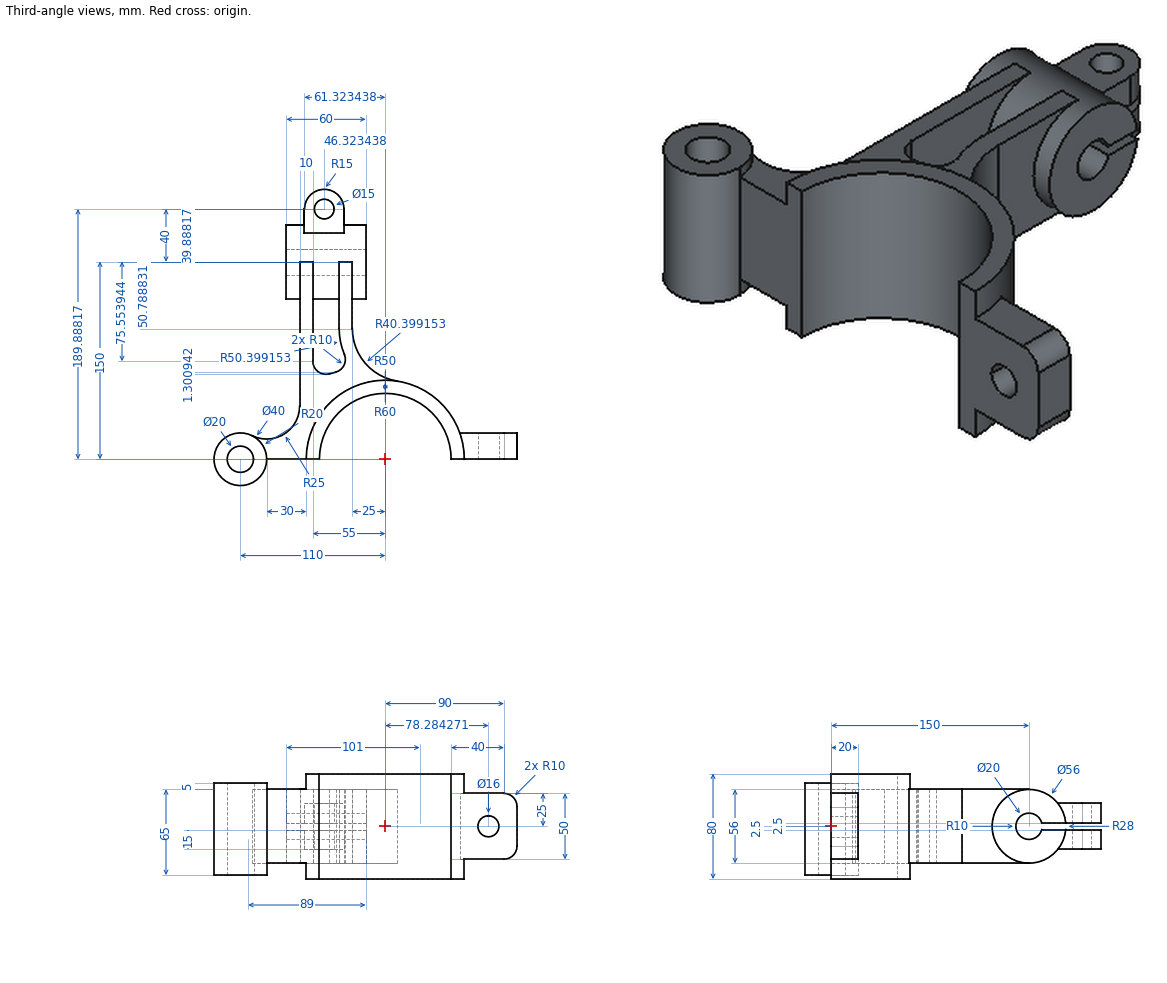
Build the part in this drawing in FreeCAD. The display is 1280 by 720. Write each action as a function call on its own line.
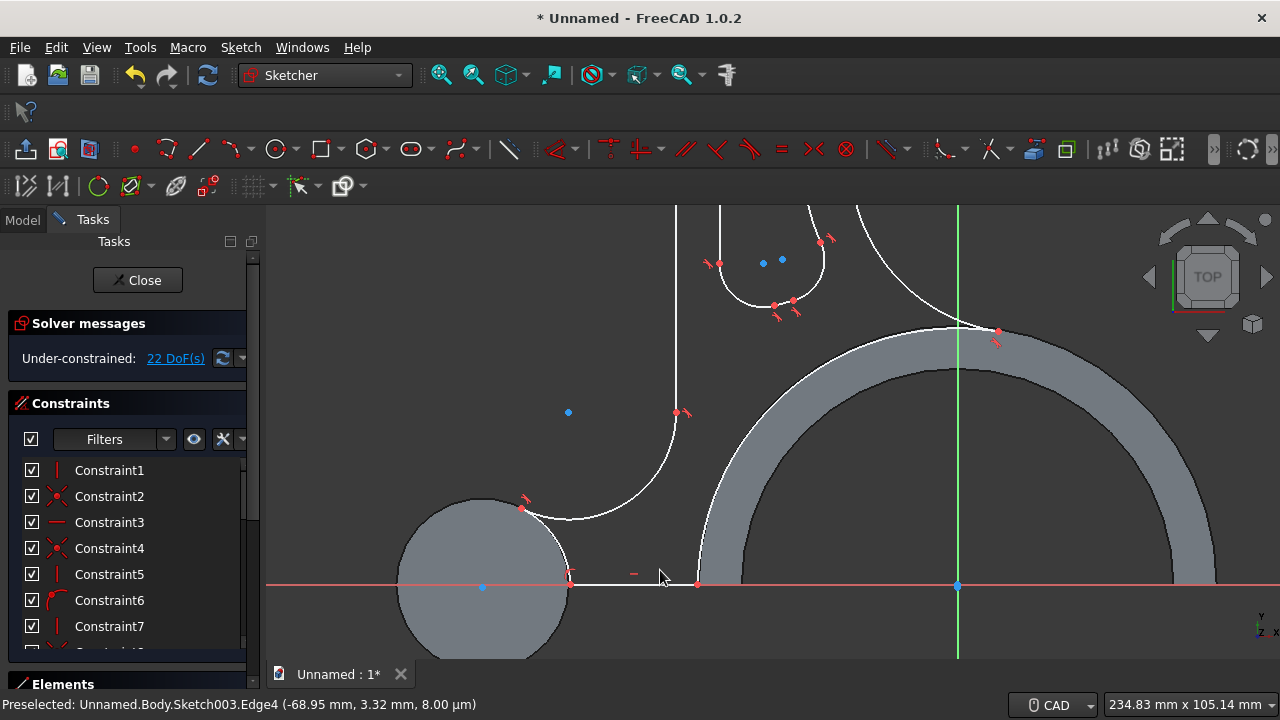
click(929, 305)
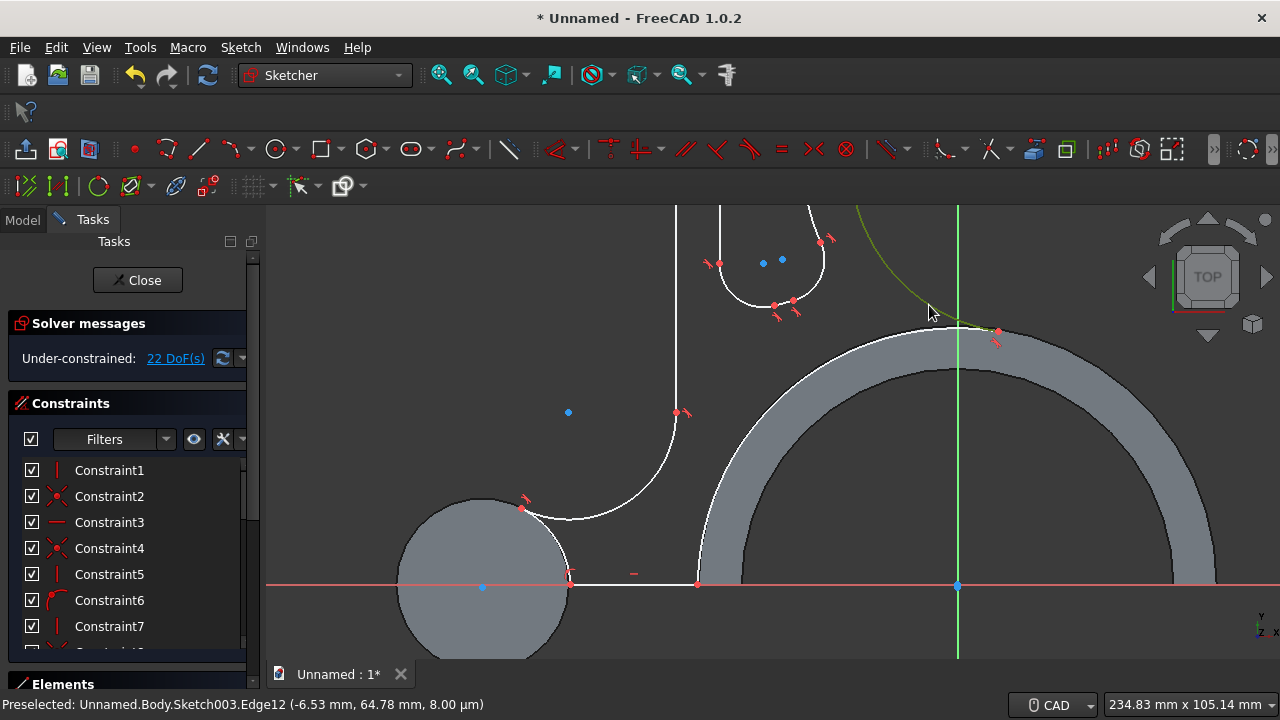
scroll(660, 572, down, 4)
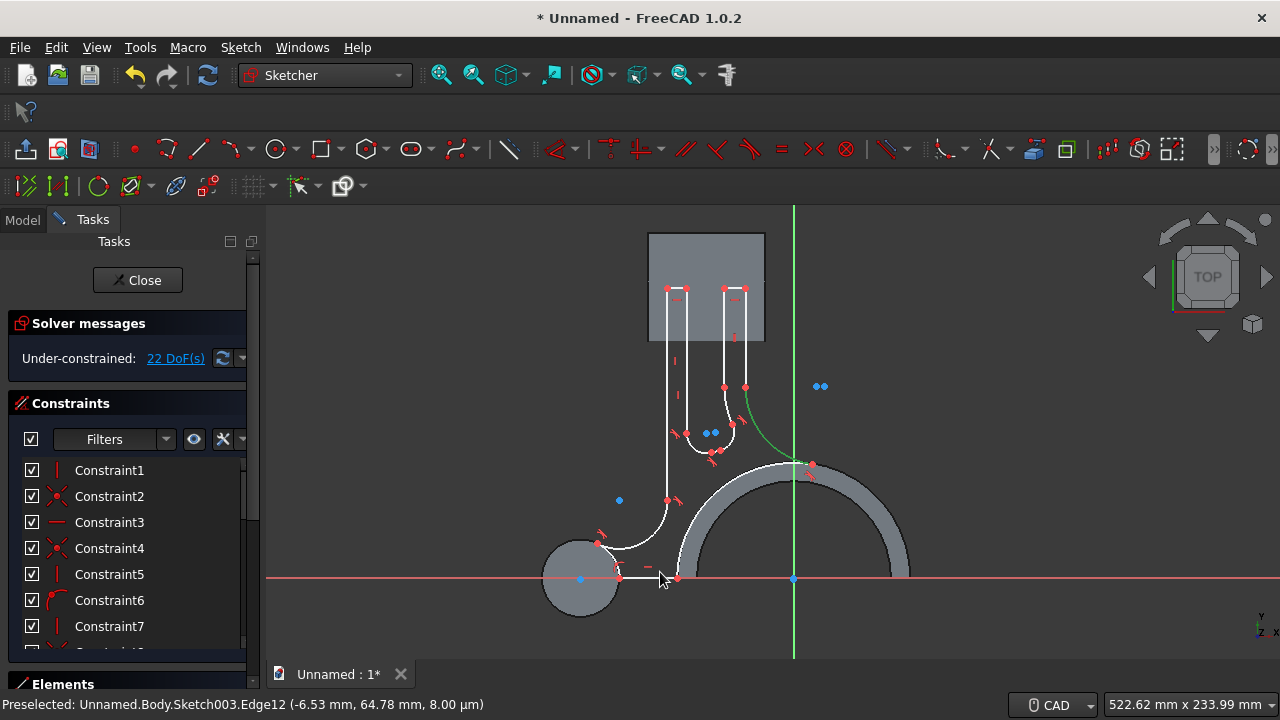
click(725, 399)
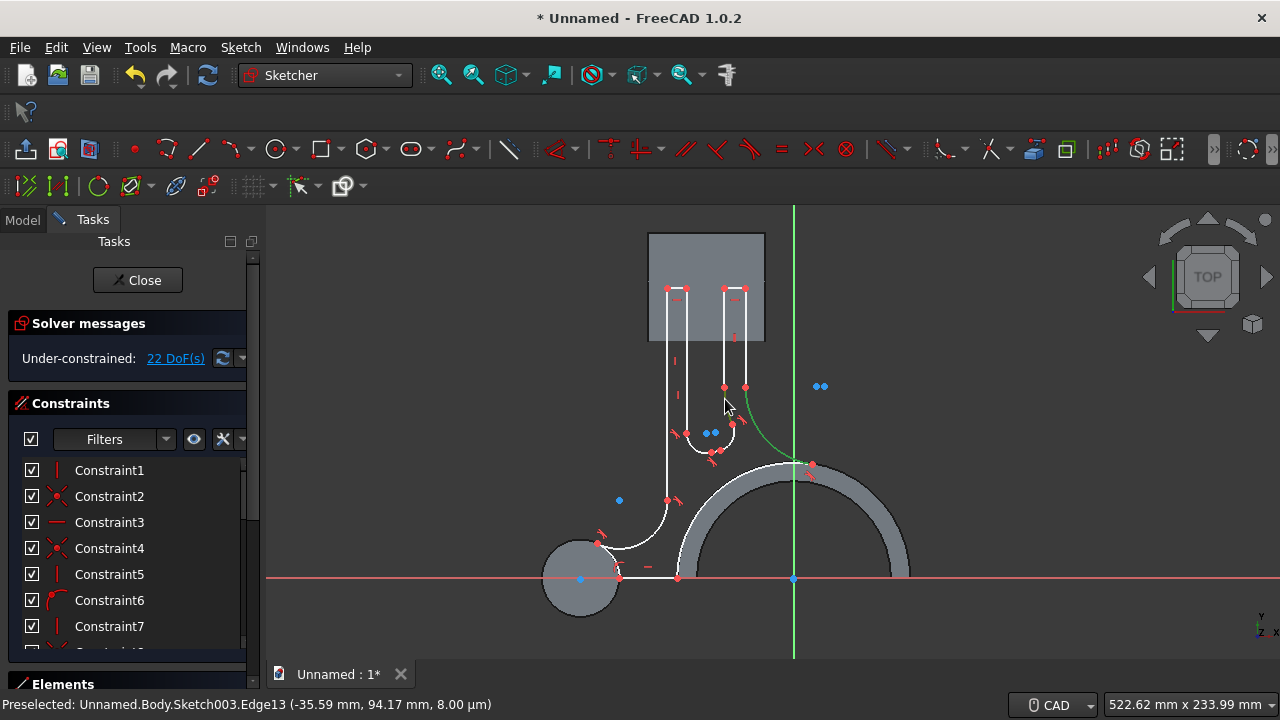
key(c)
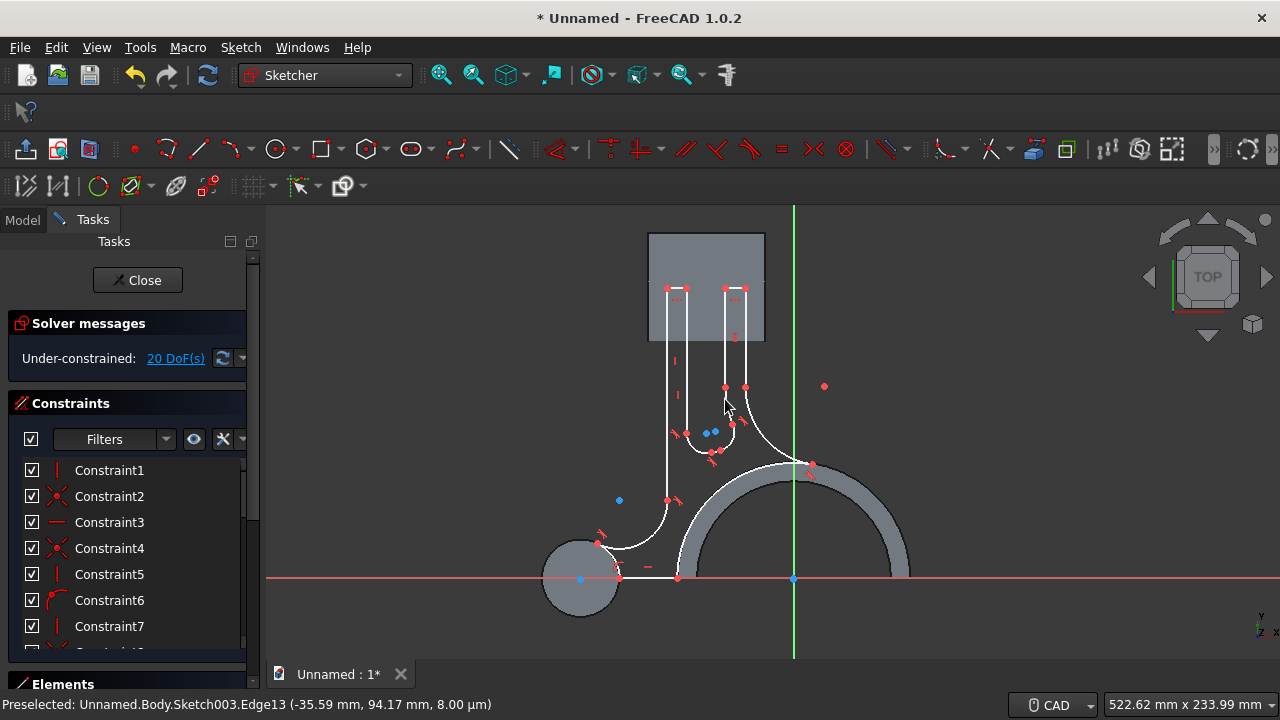
scroll(794, 579, up, 4)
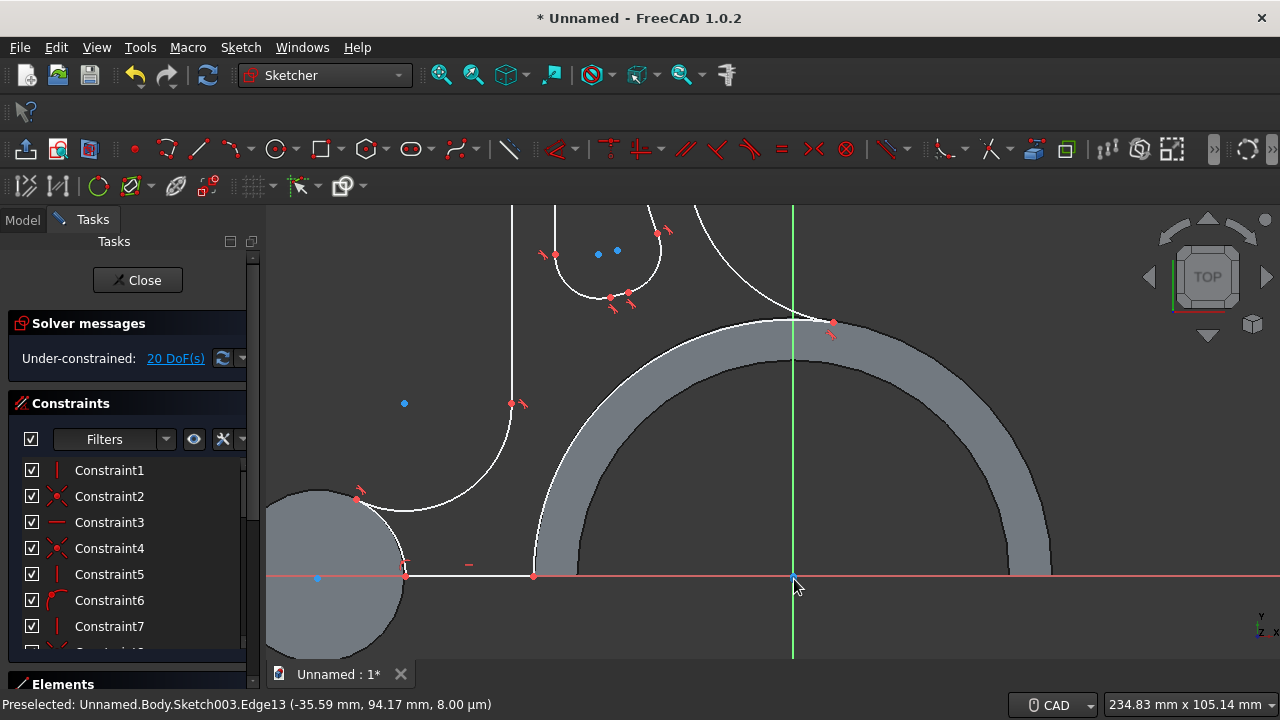
drag(783, 566, 803, 589)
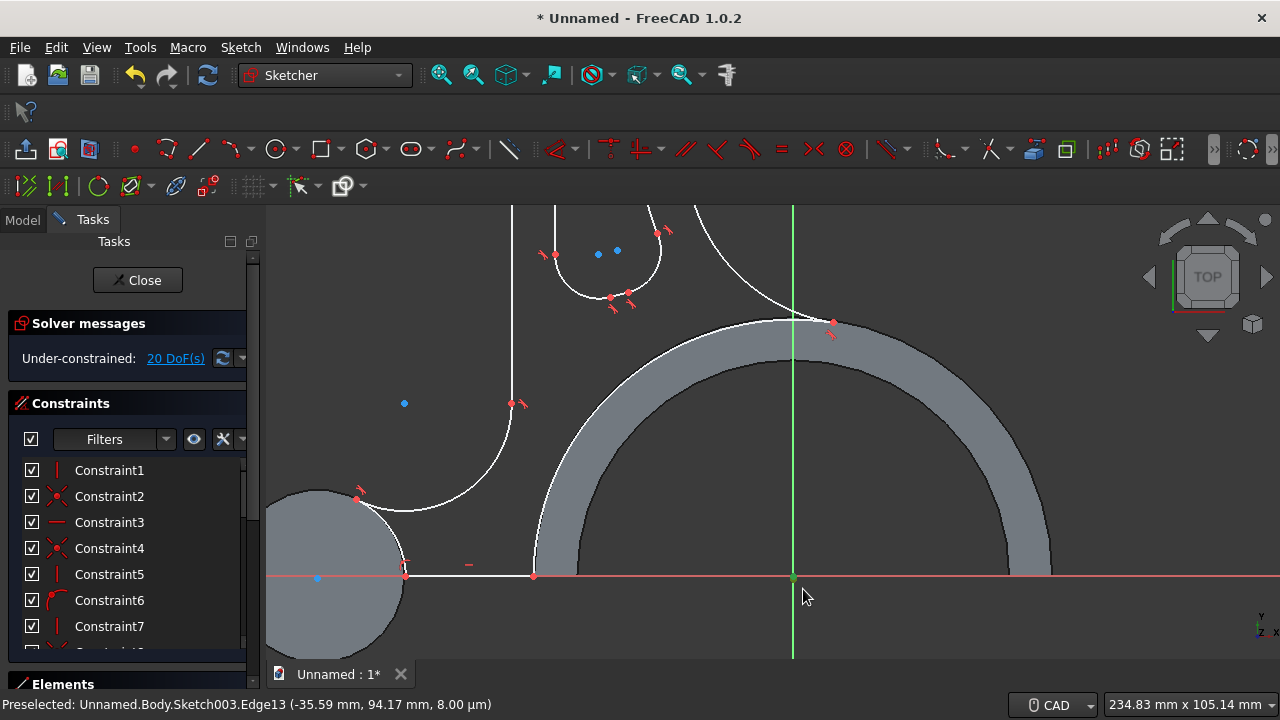
click(610, 150)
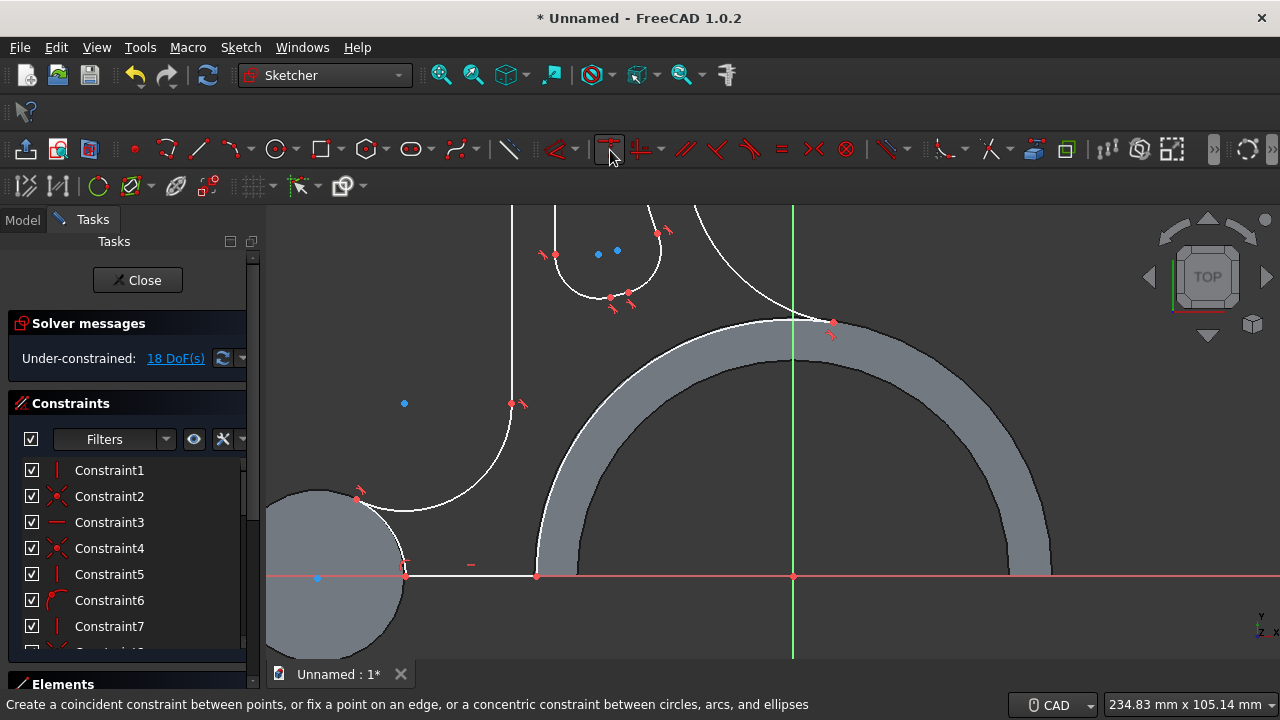
click(648, 281)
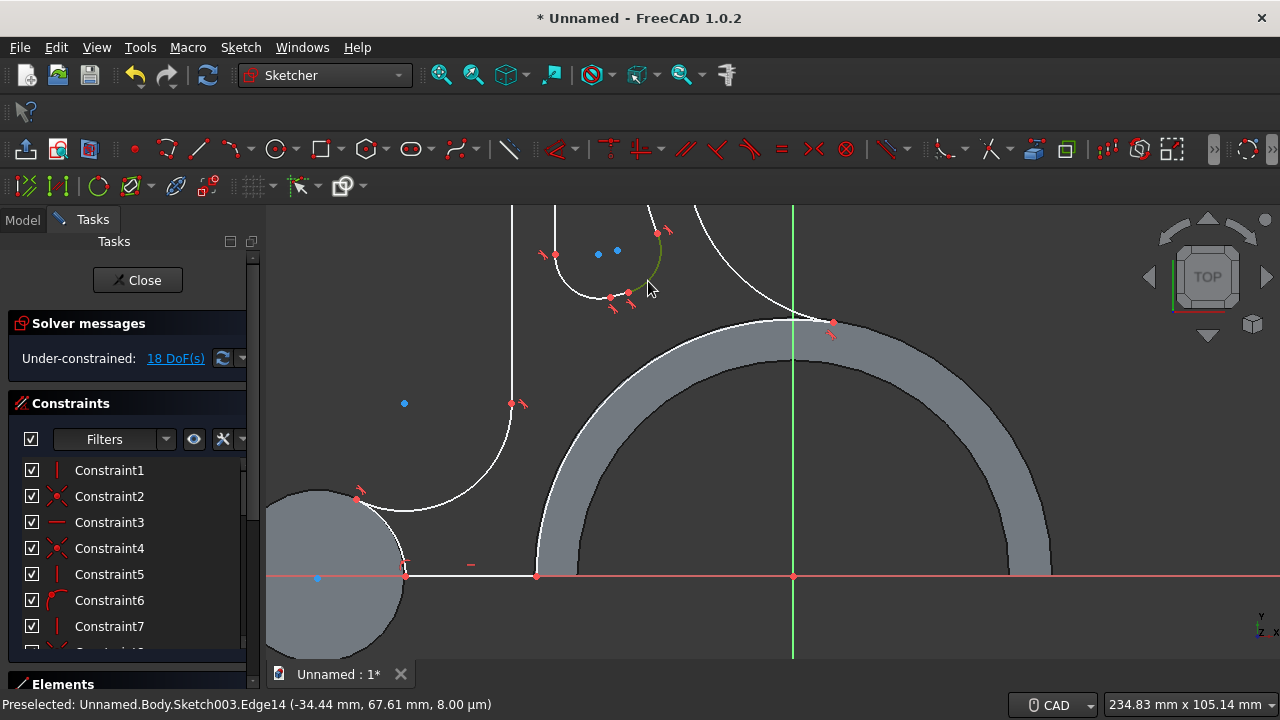
click(562, 278)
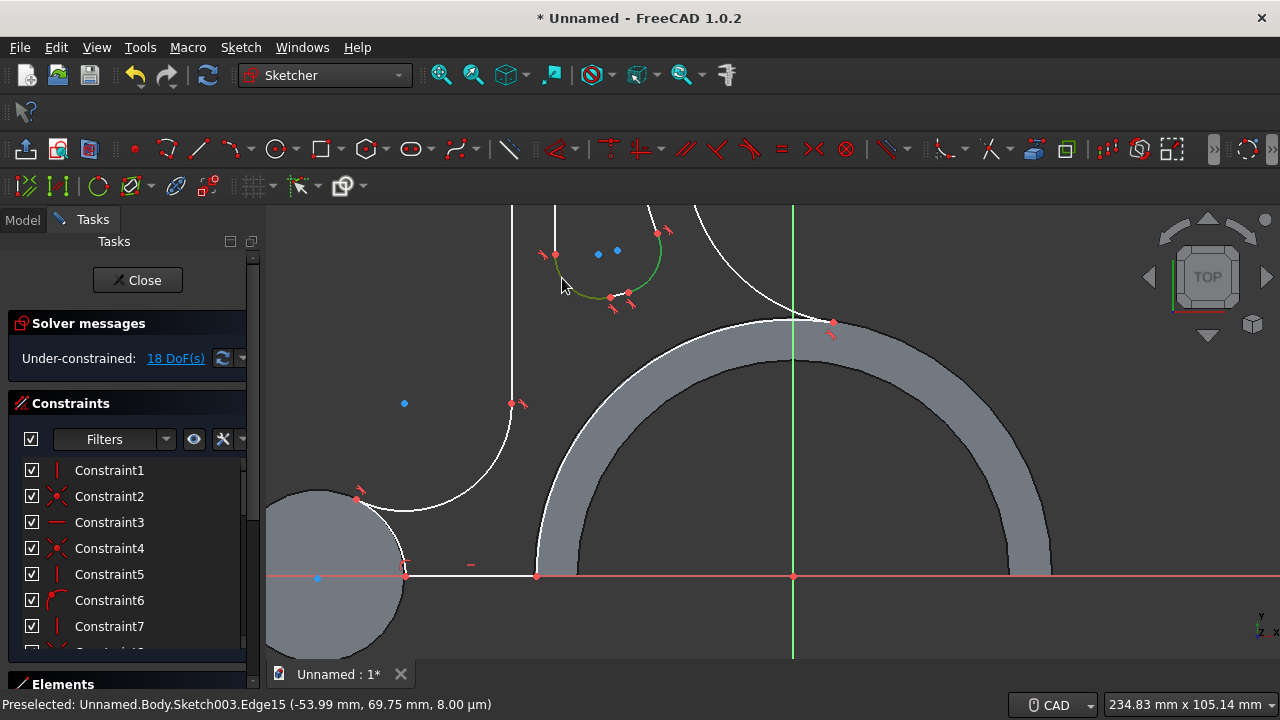
click(782, 150)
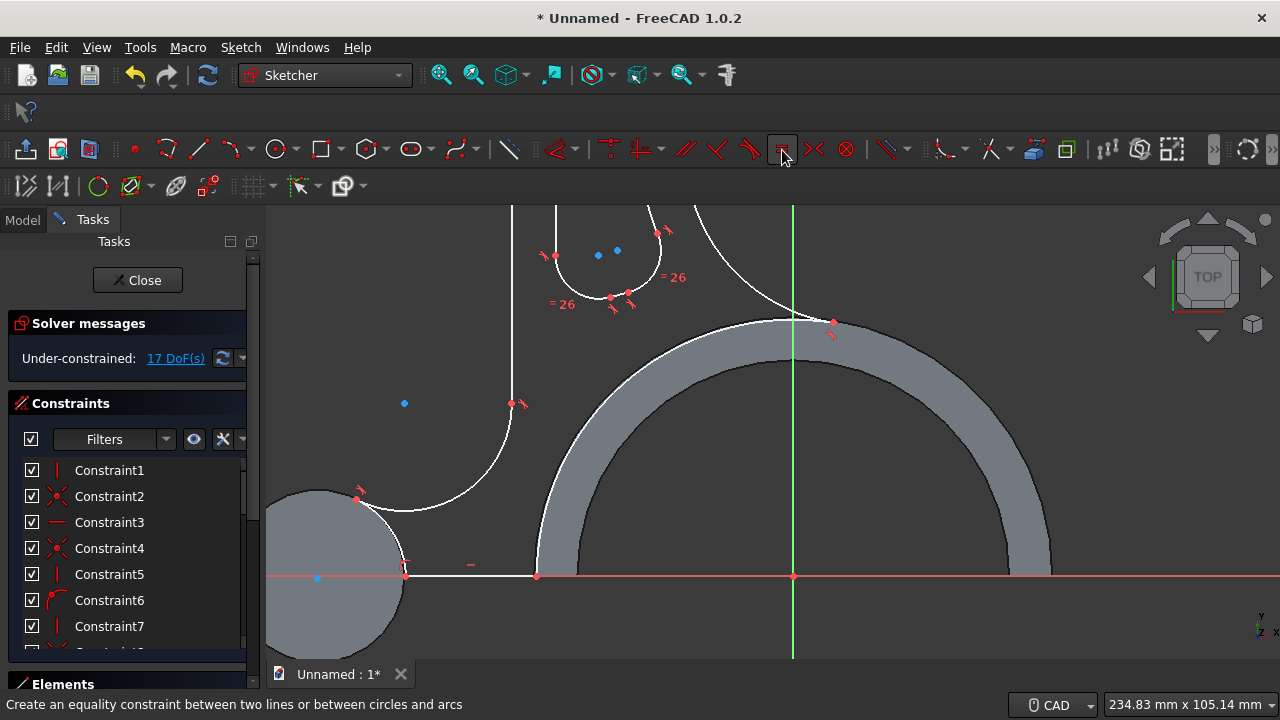
click(318, 579)